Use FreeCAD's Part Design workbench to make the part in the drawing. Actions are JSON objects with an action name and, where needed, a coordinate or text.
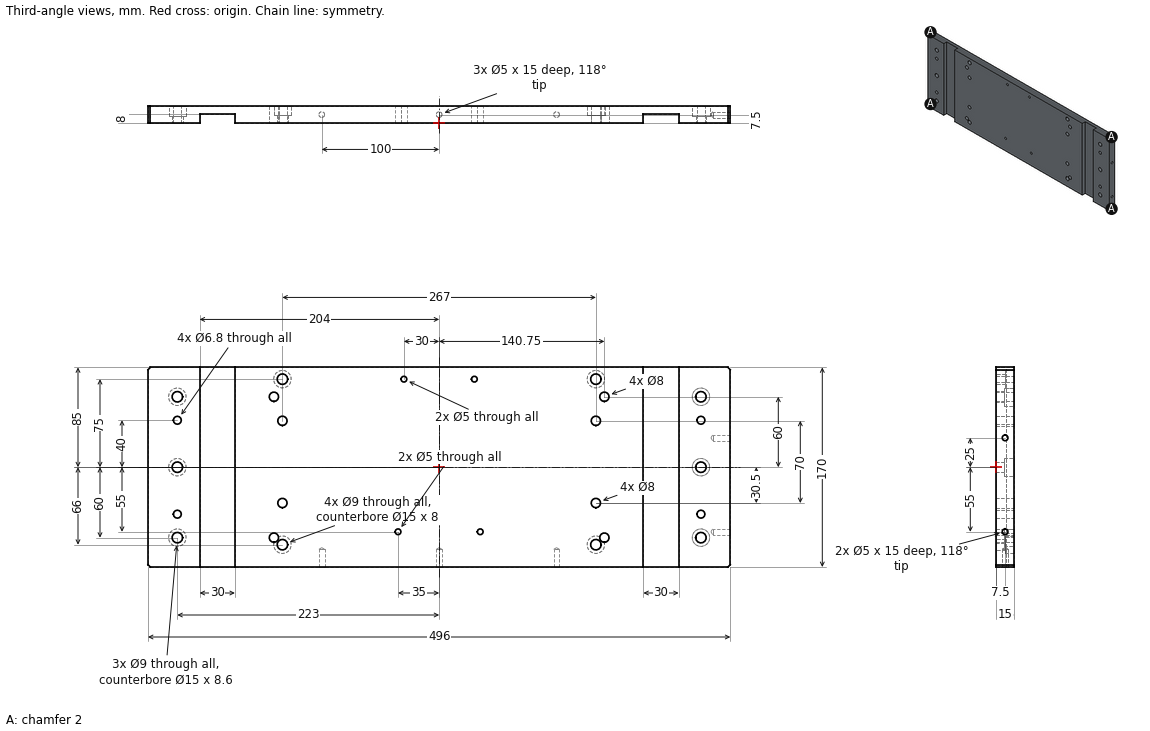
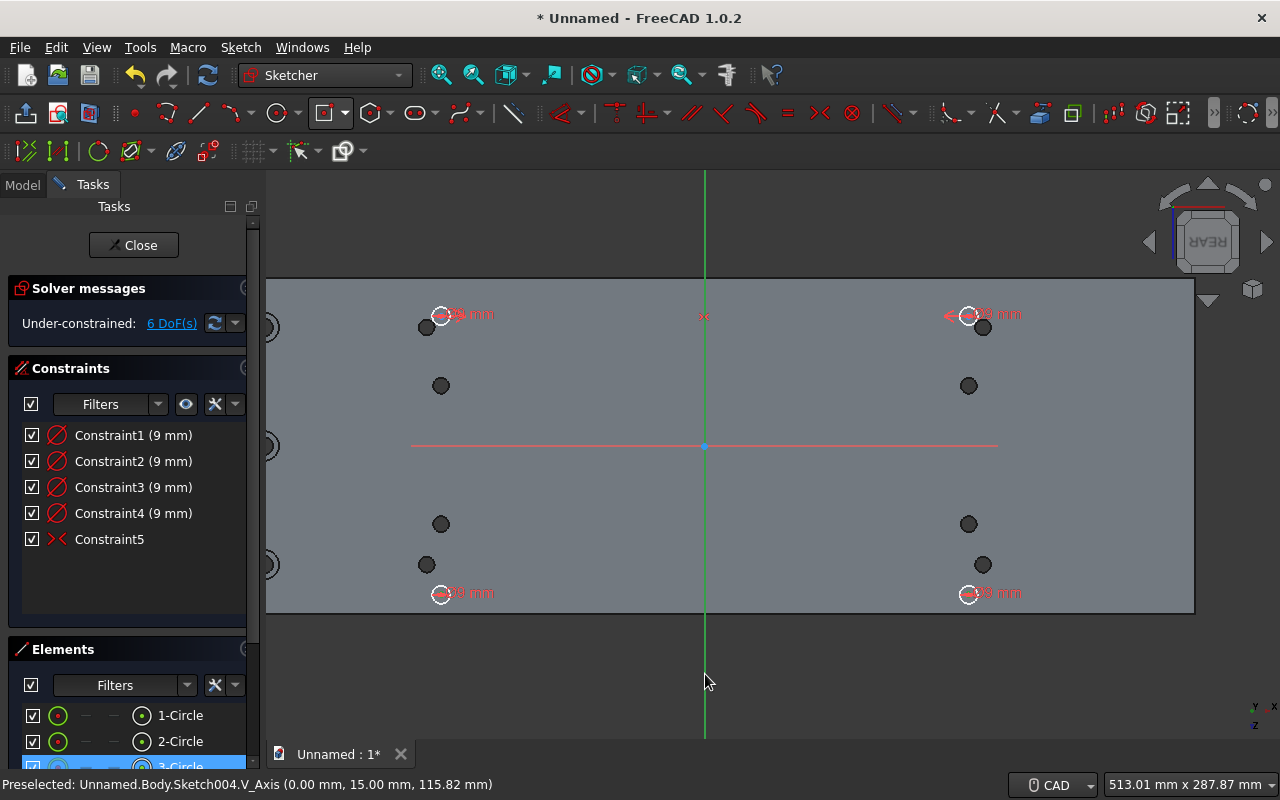
{"action": "left_click", "coordinate": [820, 114]}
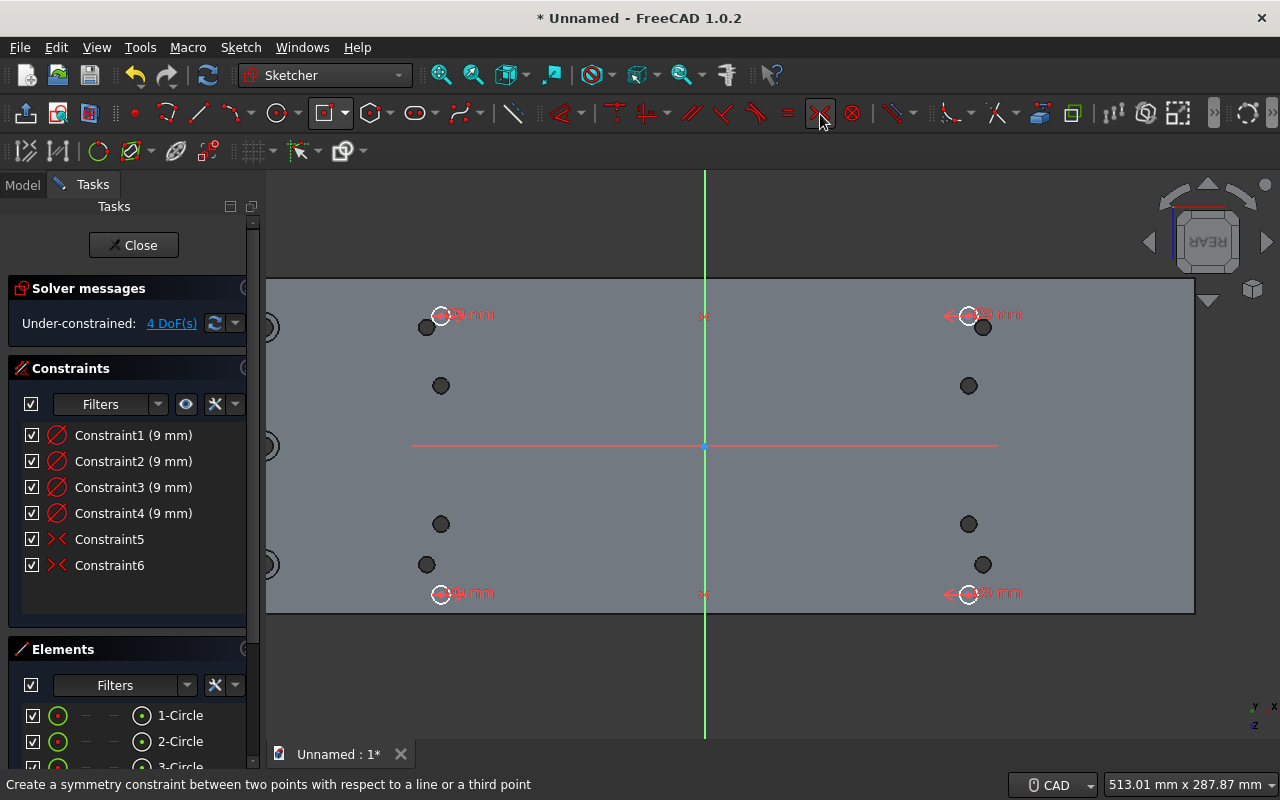
{"action": "left_click", "coordinate": [560, 114]}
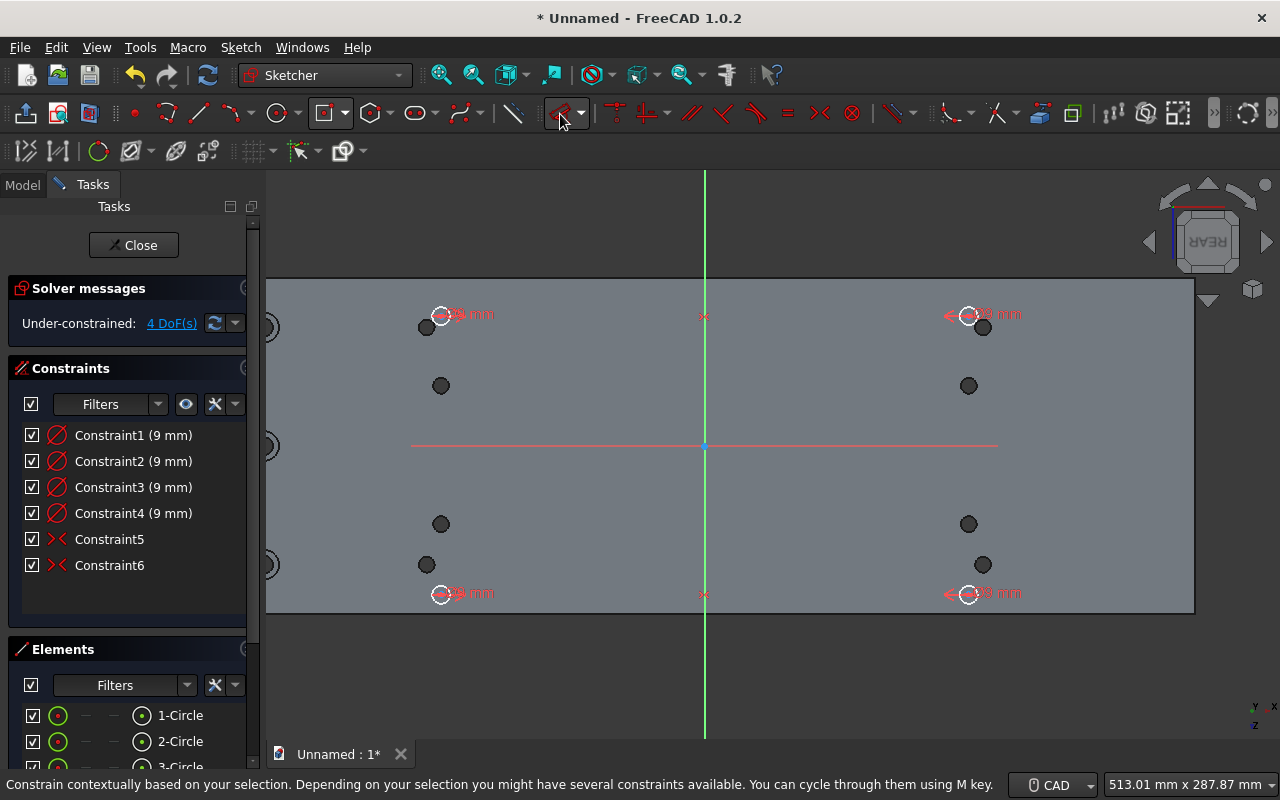
{"action": "left_click", "coordinate": [441, 316]}
{"action": "left_click", "coordinate": [407, 381]}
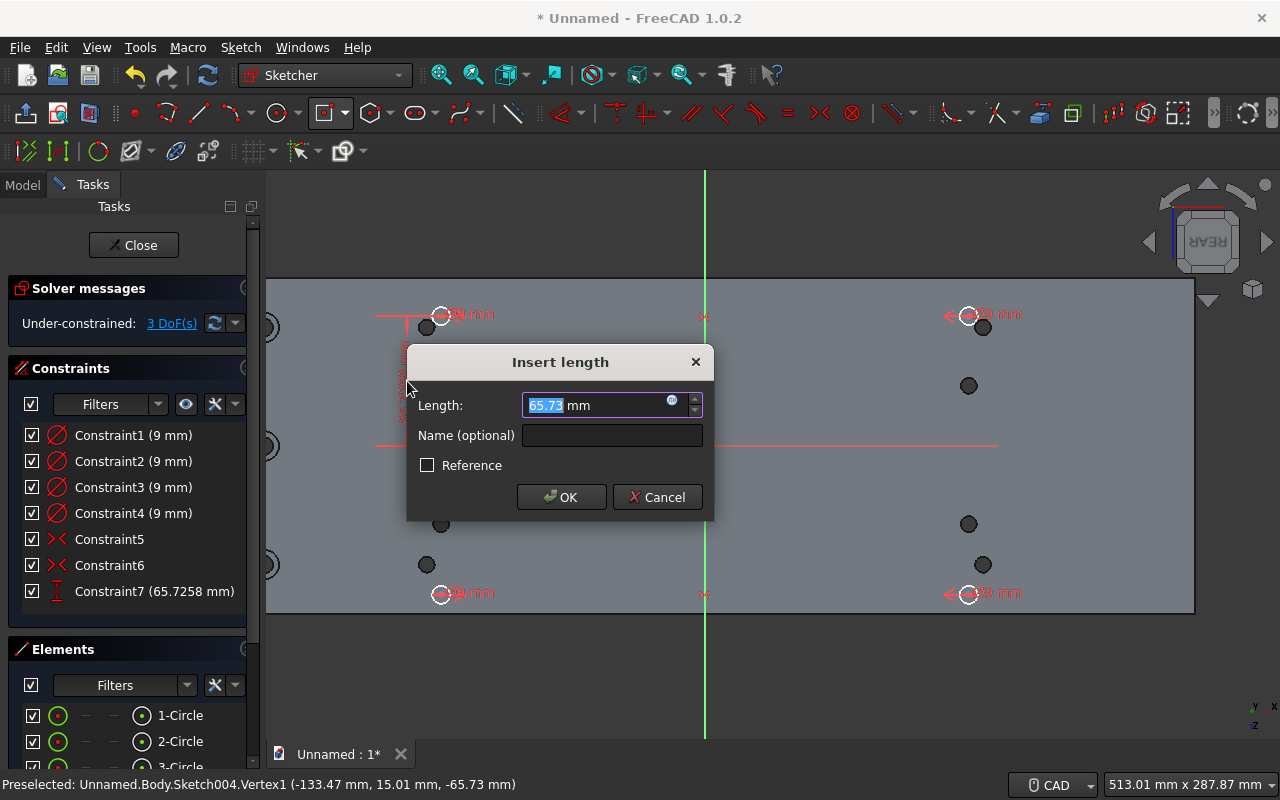
{"action": "type", "text": "66"}
{"action": "key", "text": "Return"}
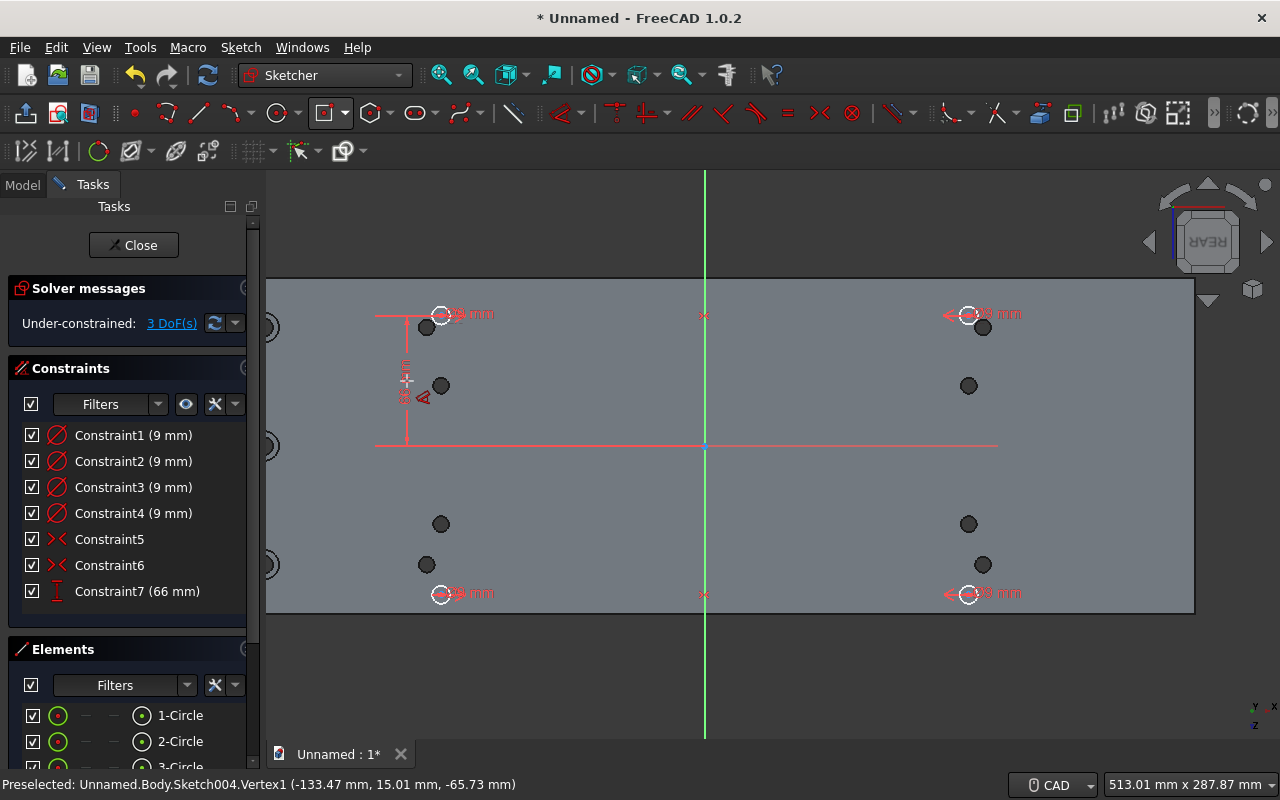
{"action": "left_click", "coordinate": [441, 595]}
{"action": "left_click", "coordinate": [407, 520]}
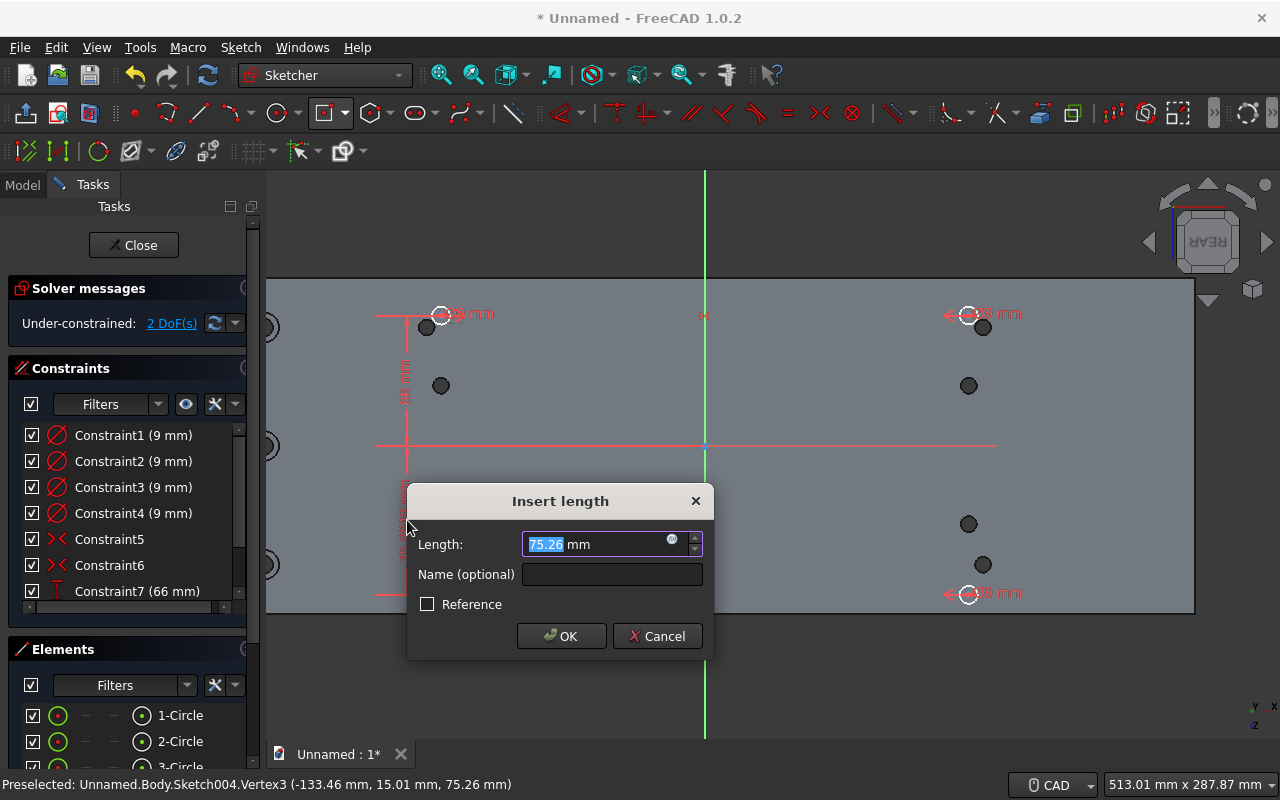
{"action": "type", "text": "75"}
{"action": "key", "text": "Return"}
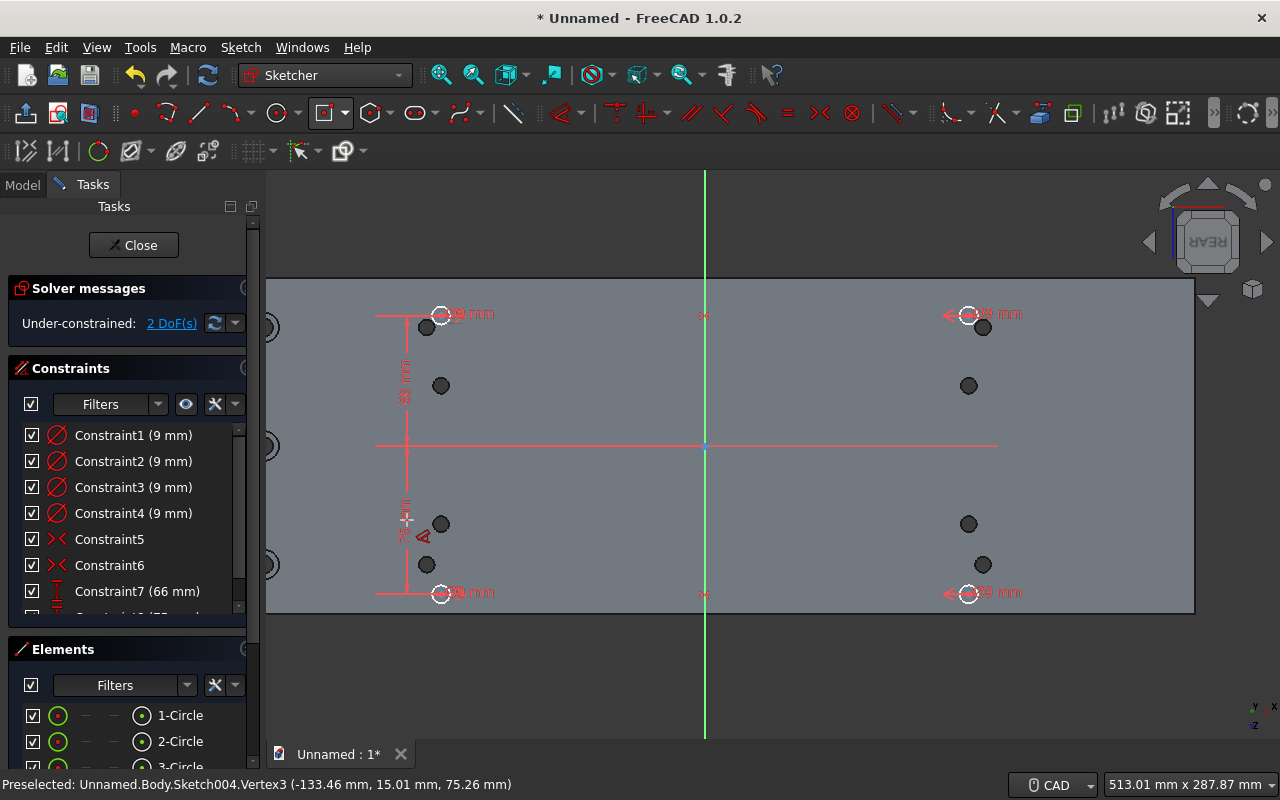
{"action": "left_click", "coordinate": [441, 316]}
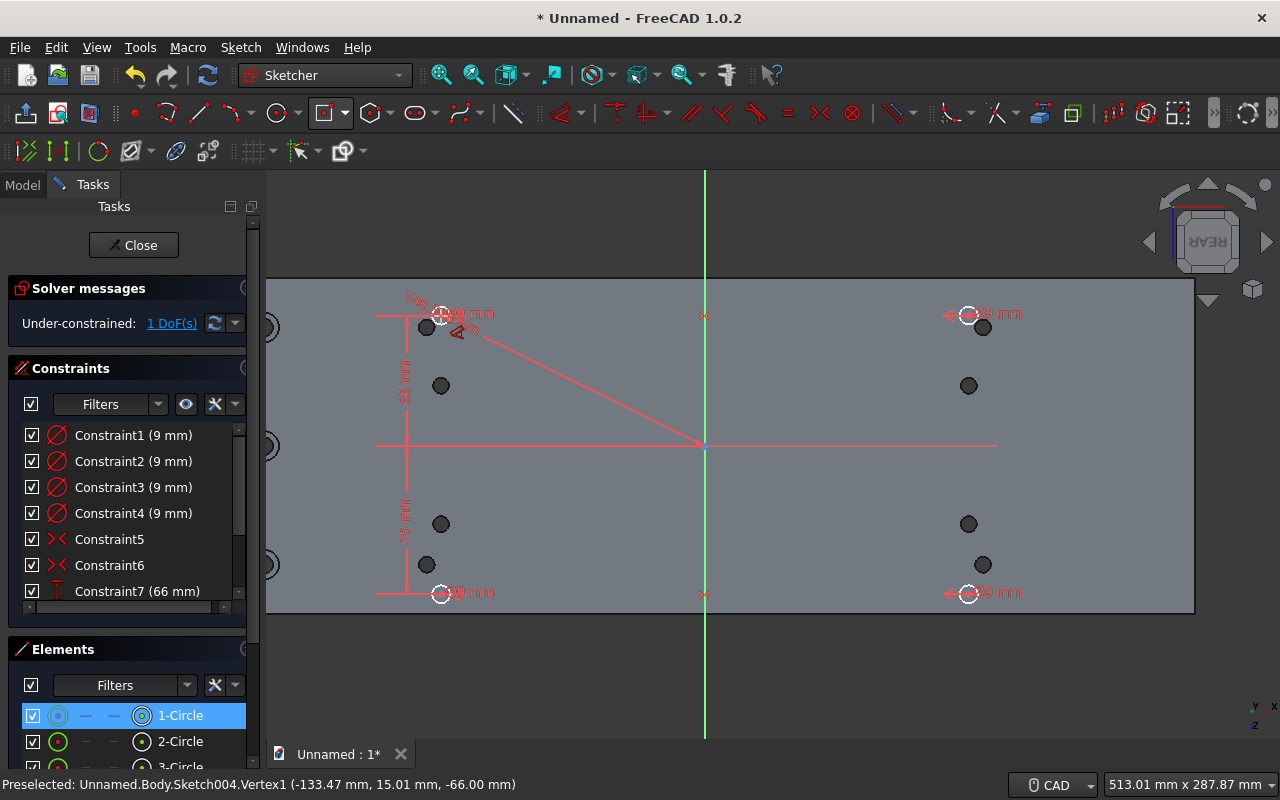
{"action": "left_click", "coordinate": [969, 316]}
{"action": "left_click", "coordinate": [584, 282]}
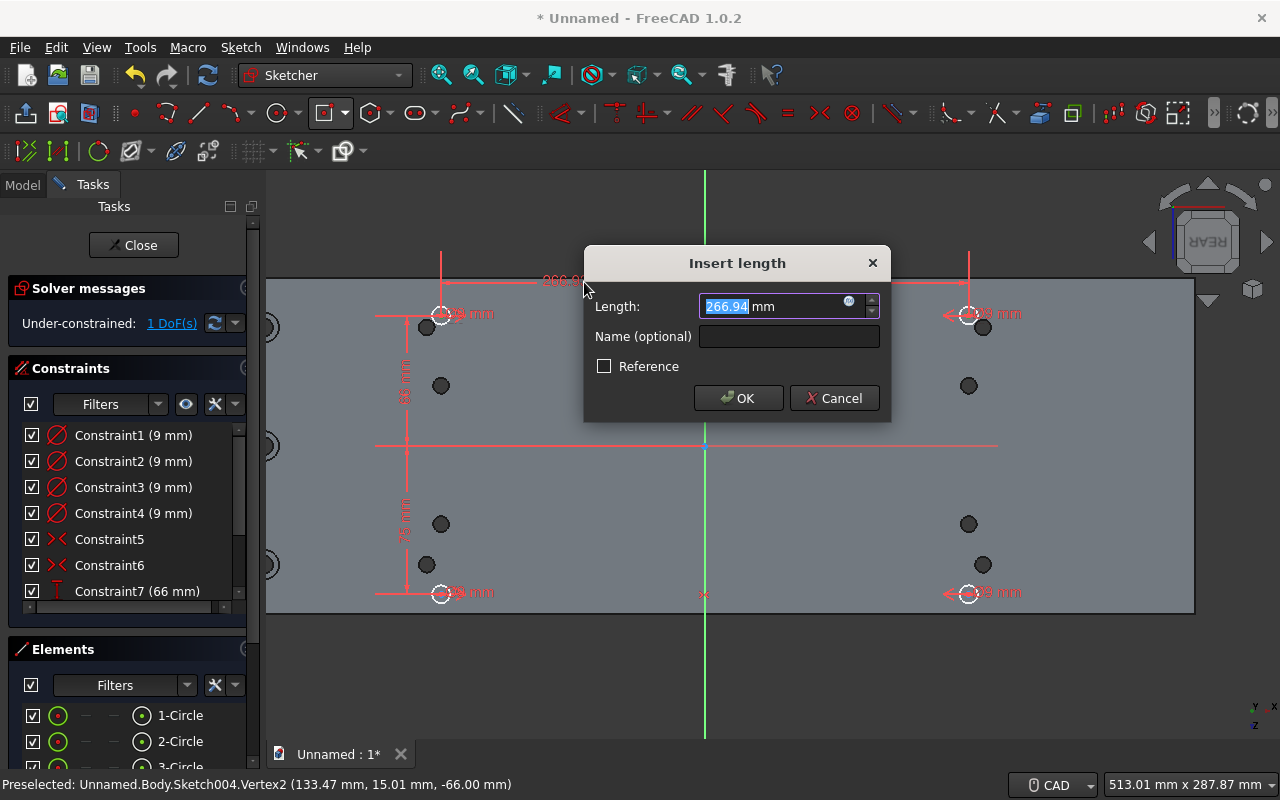
{"action": "type", "text": "267"}
{"action": "key", "text": "Return"}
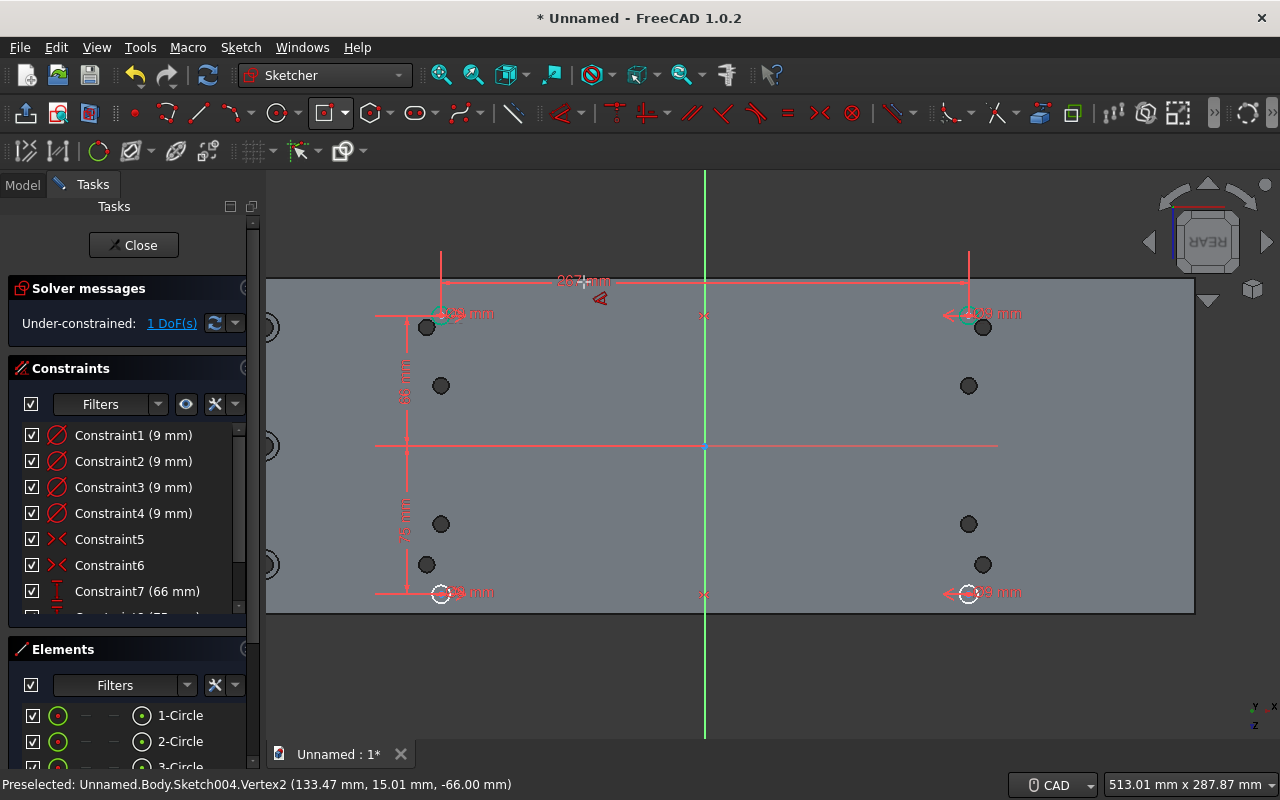
{"action": "left_click", "coordinate": [969, 316]}